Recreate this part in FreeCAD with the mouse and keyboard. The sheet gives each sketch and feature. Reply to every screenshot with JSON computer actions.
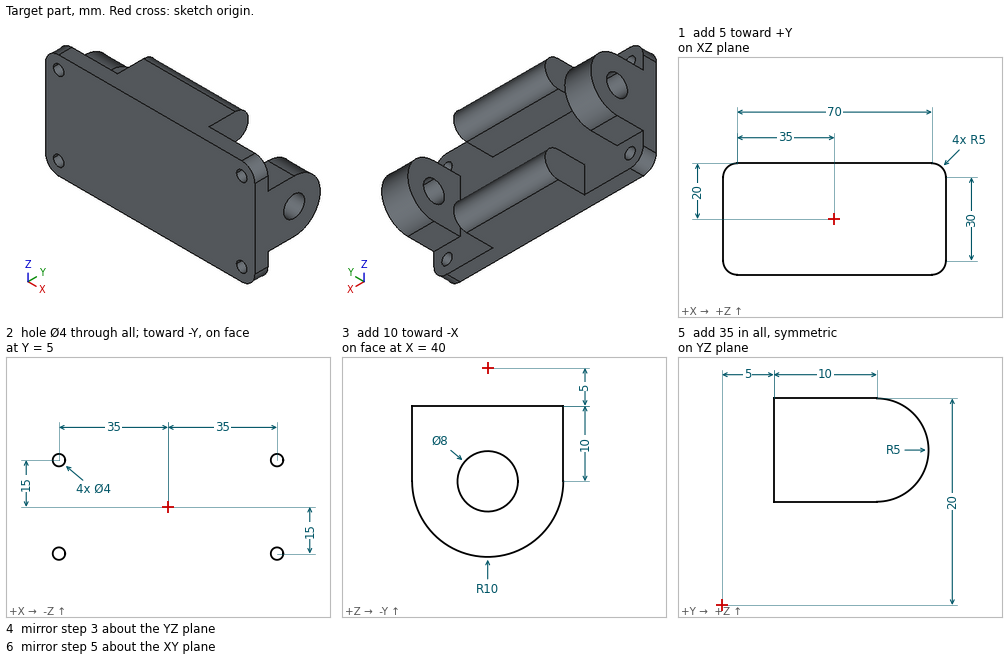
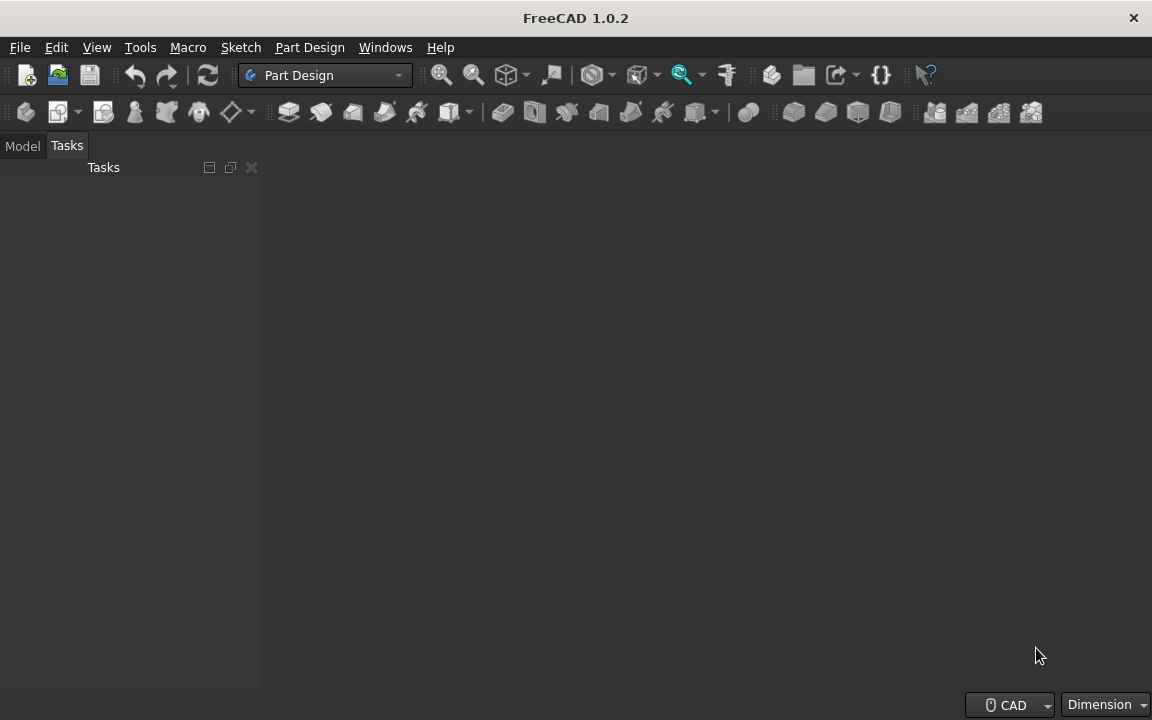
{"action": "left_click", "coordinate": [26, 76]}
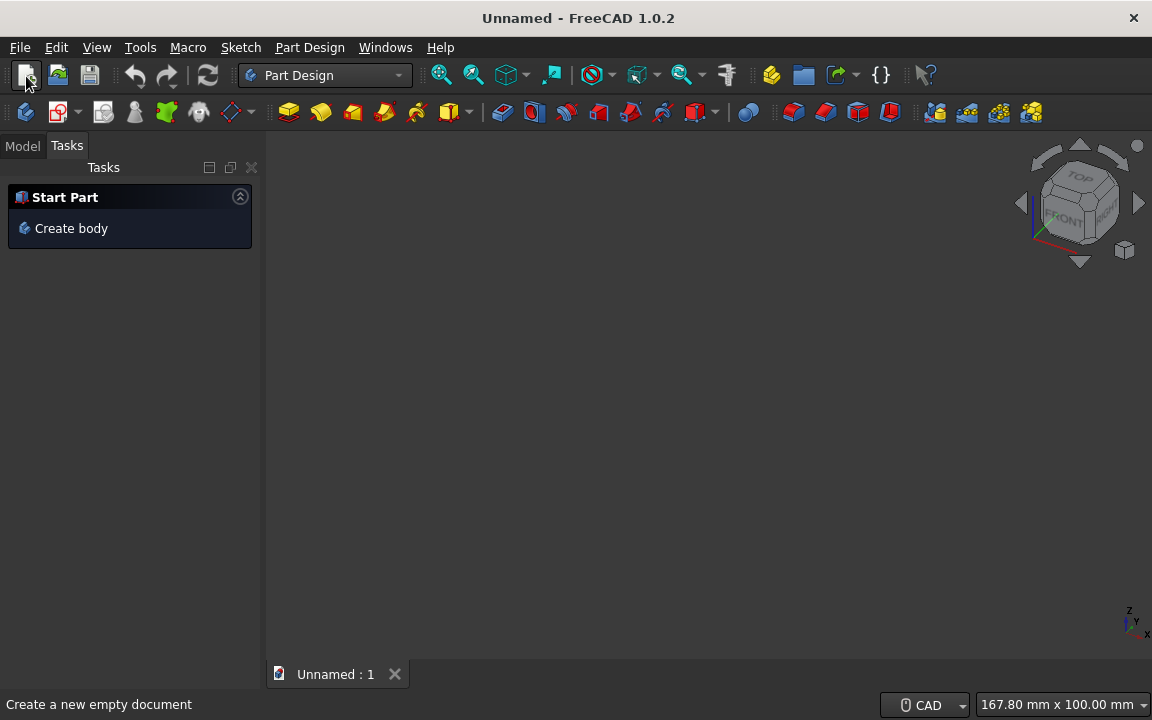
{"action": "left_click", "coordinate": [58, 112]}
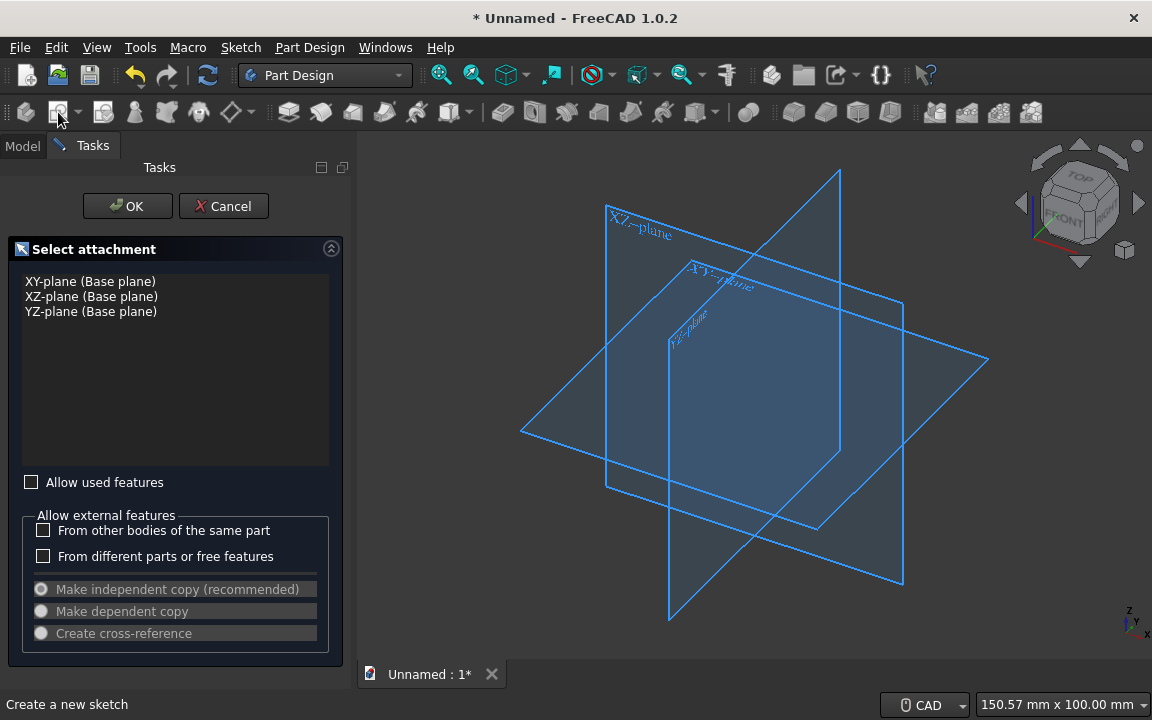
{"action": "left_click", "coordinate": [82, 296]}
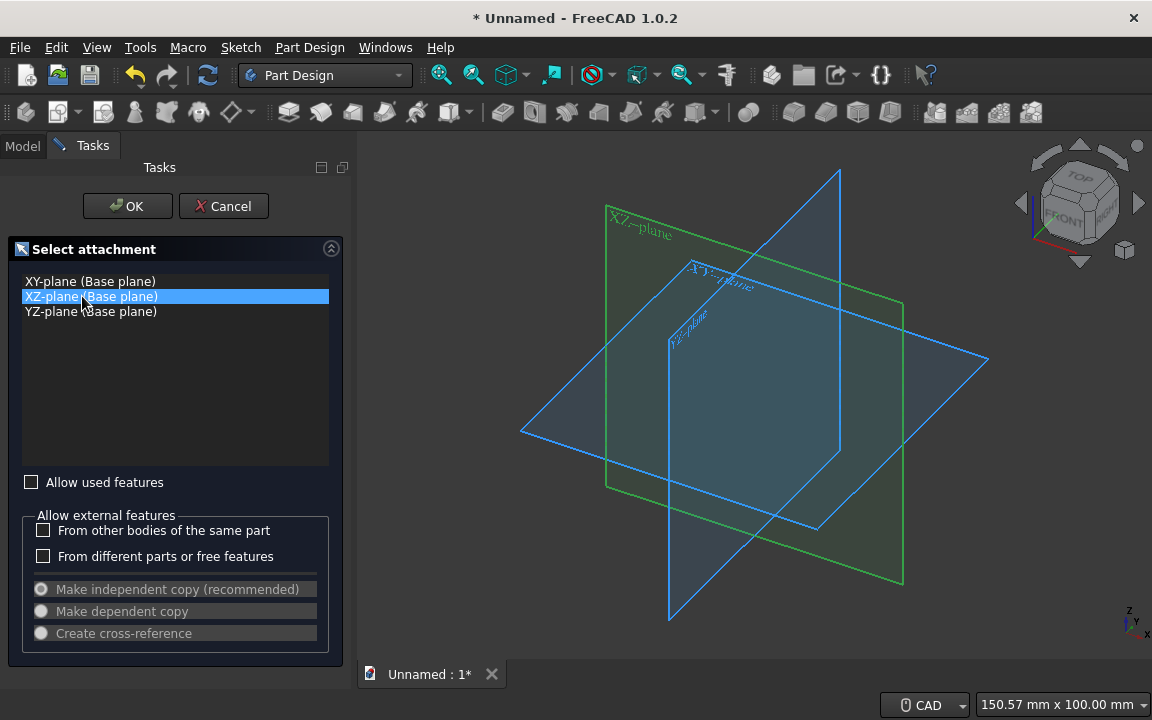
{"action": "left_click", "coordinate": [128, 206]}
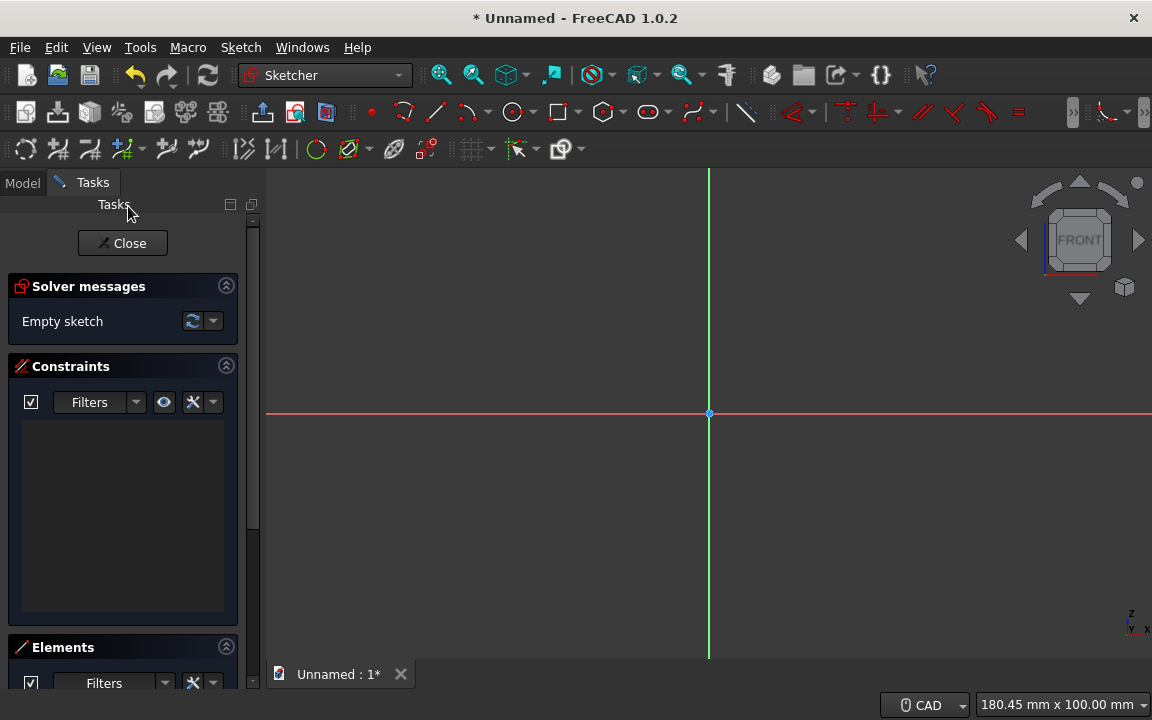
{"action": "left_click", "coordinate": [436, 112]}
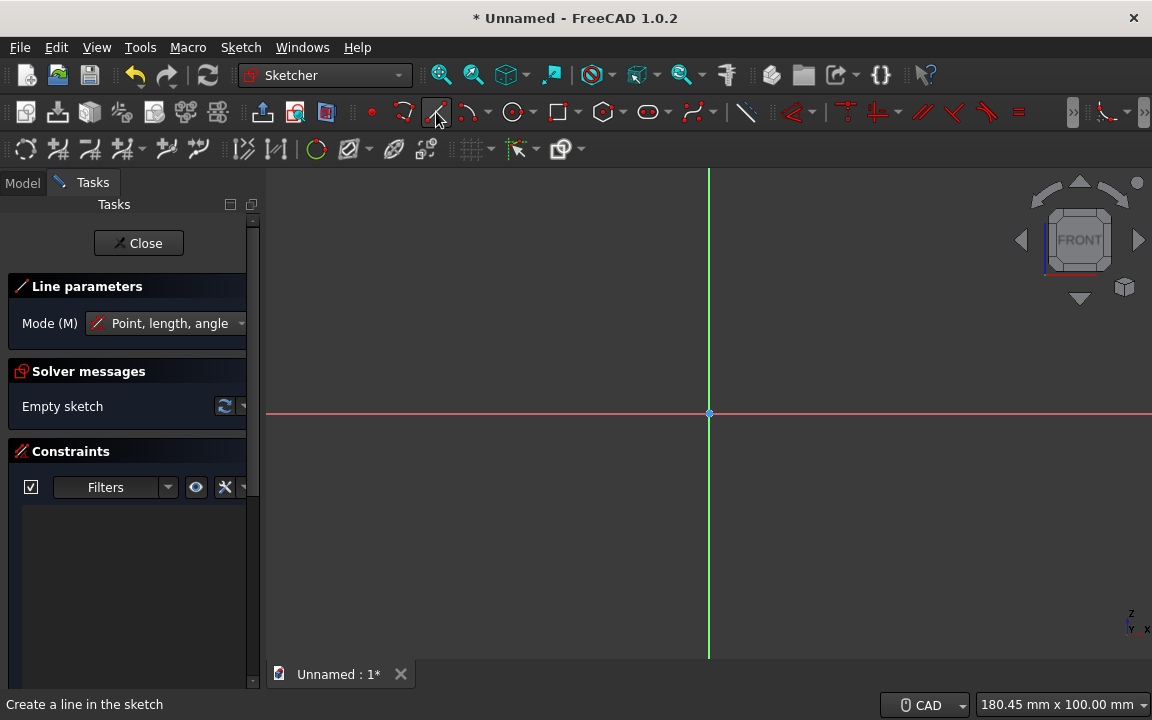
{"action": "left_click", "coordinate": [537, 315]}
{"action": "left_click", "coordinate": [881, 315]}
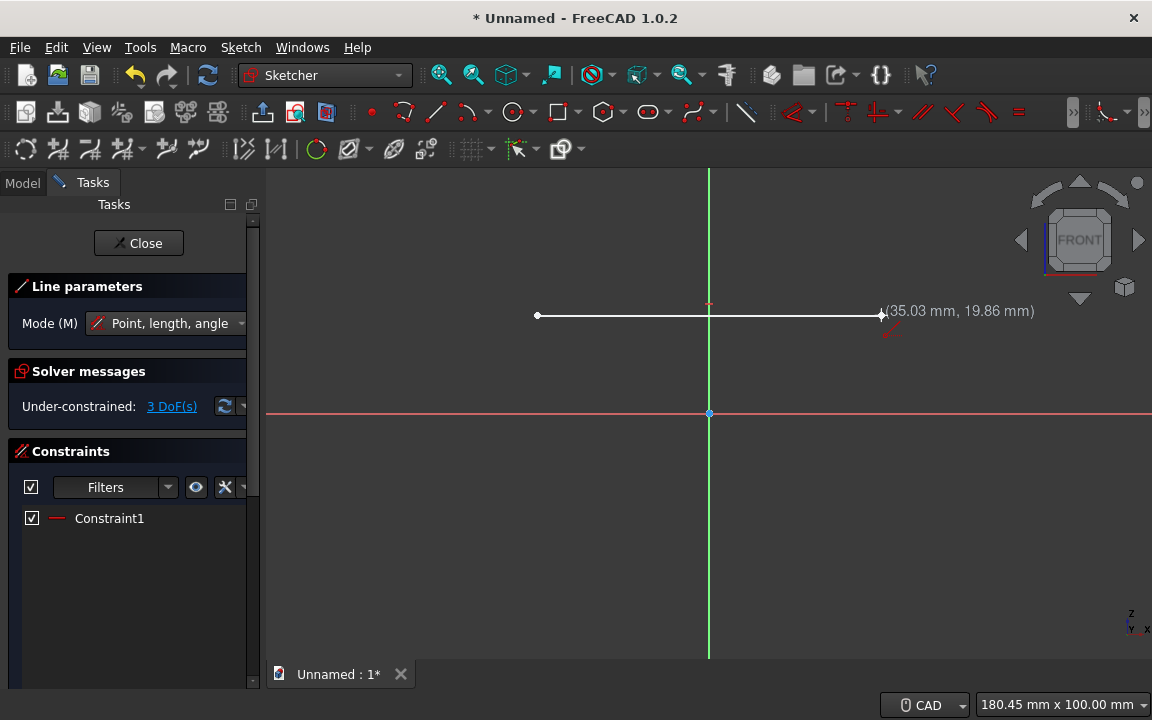
{"action": "left_click", "coordinate": [905, 340]}
{"action": "left_click", "coordinate": [905, 487]}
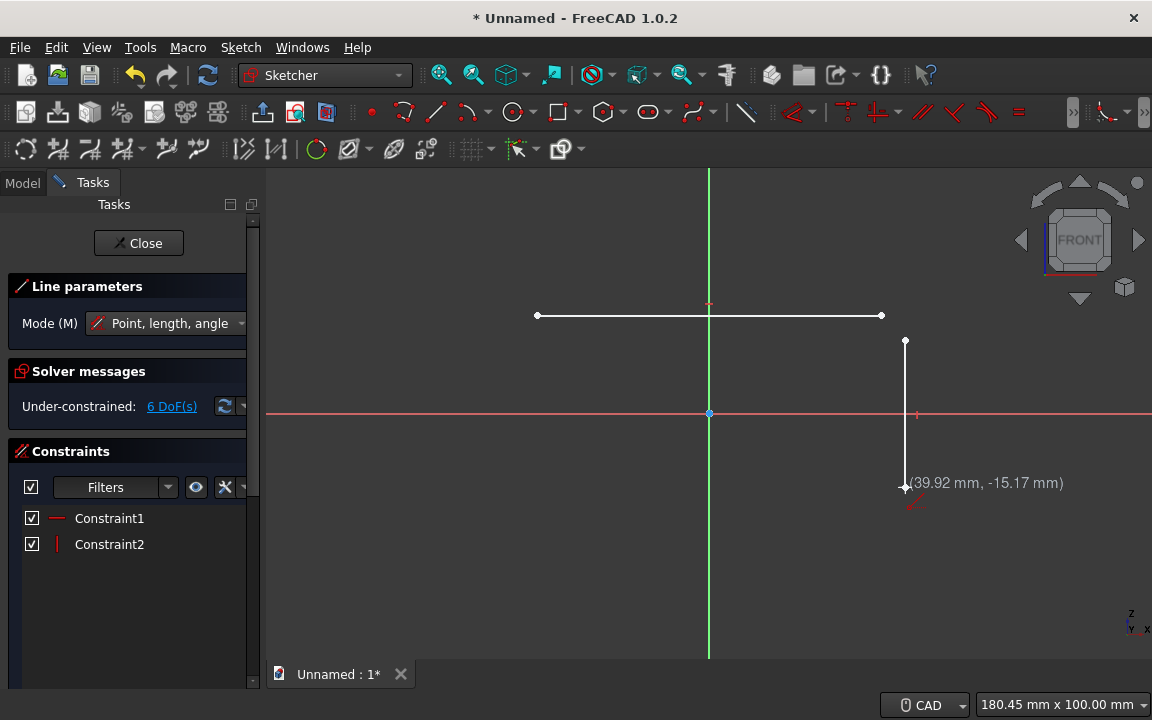
{"action": "left_click", "coordinate": [881, 512]}
{"action": "left_click", "coordinate": [537, 512]}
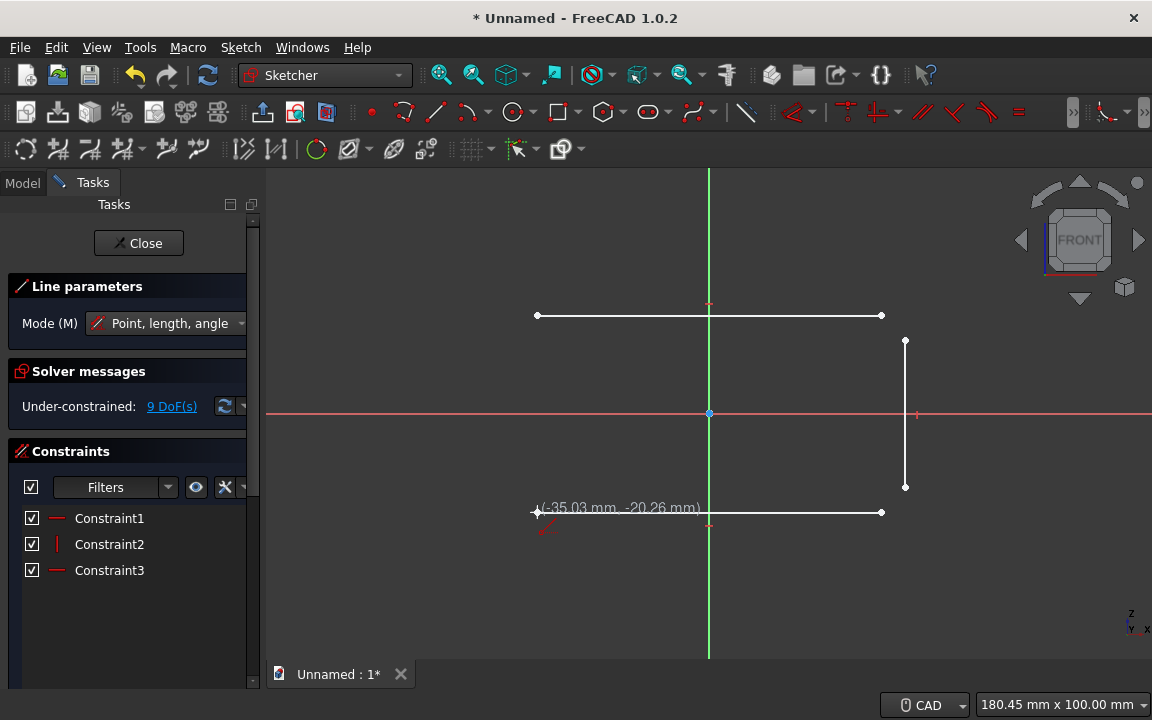
{"action": "left_click", "coordinate": [513, 487]}
{"action": "left_click", "coordinate": [513, 340]}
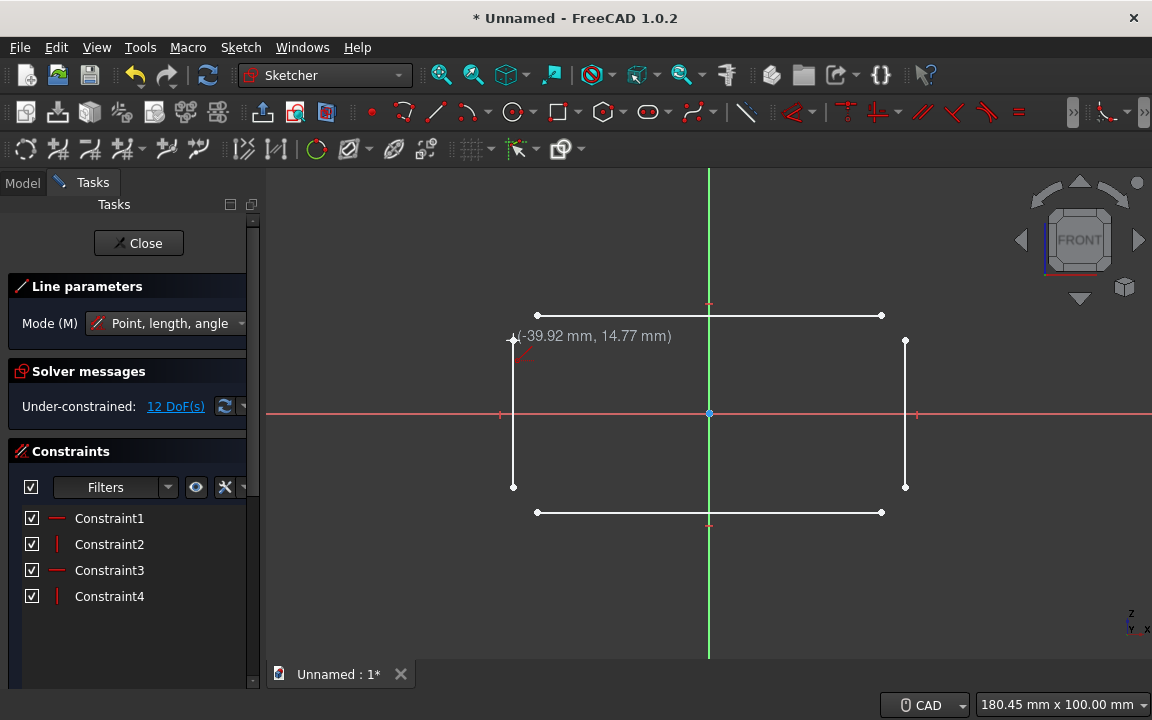
{"action": "key", "text": "g 3 a"}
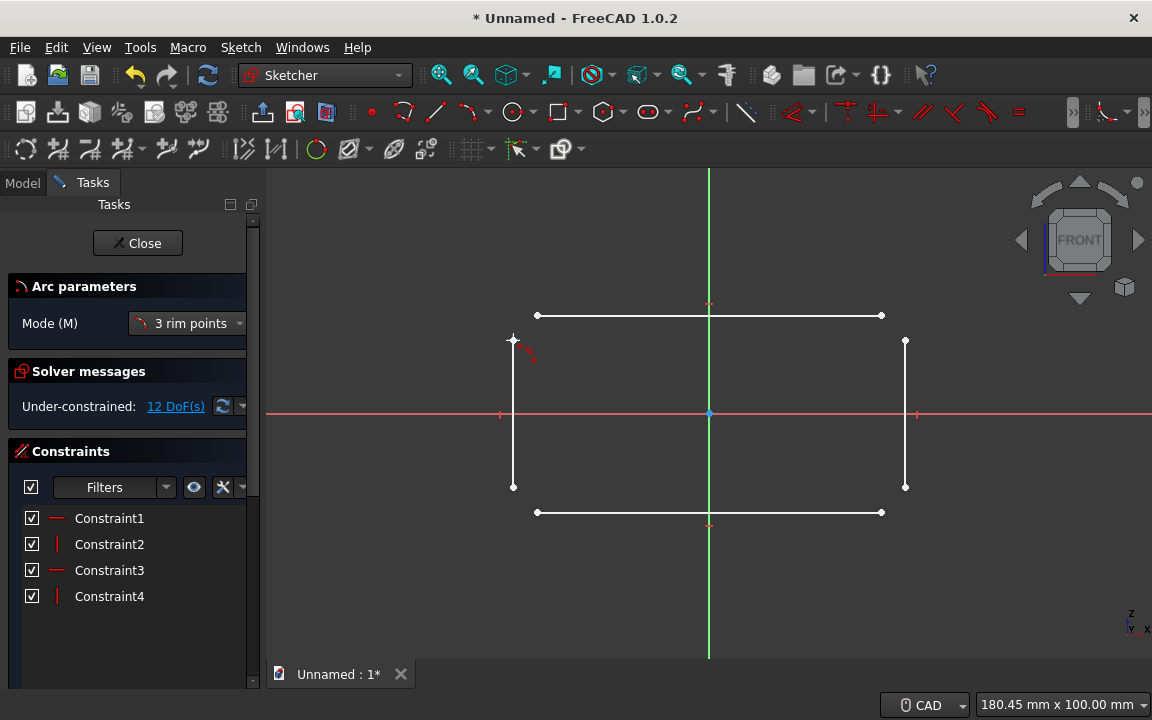
{"action": "left_click", "coordinate": [881, 316]}
{"action": "left_click", "coordinate": [905, 341]}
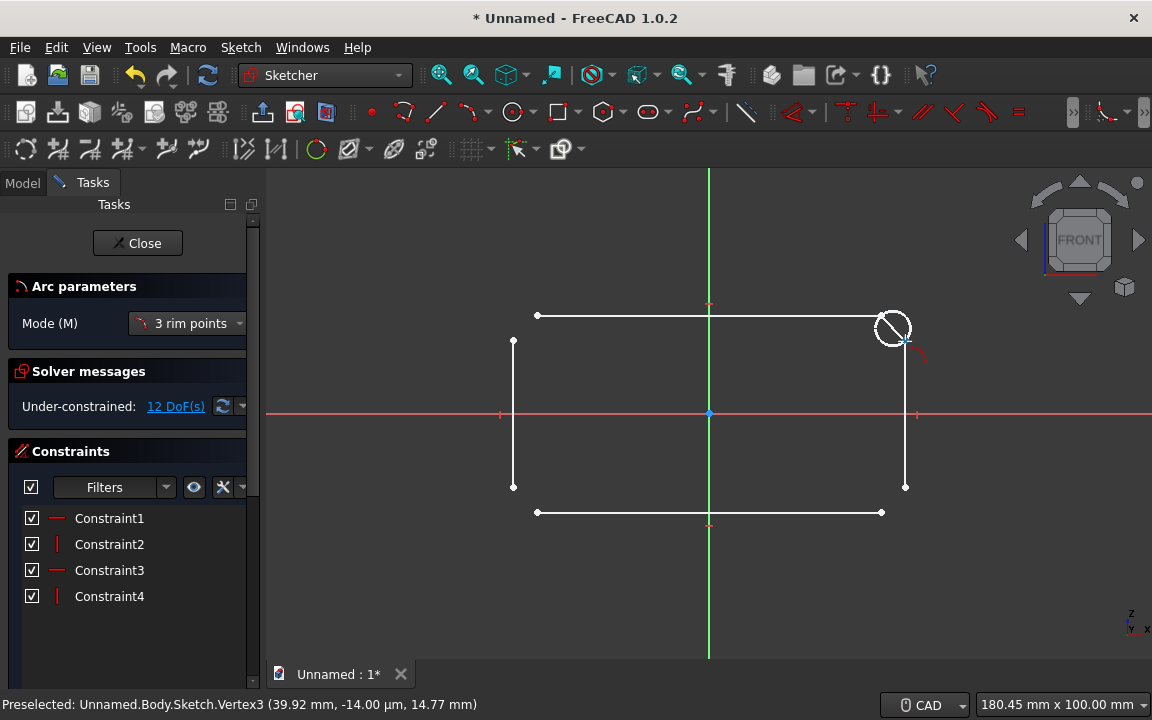
{"action": "scroll", "coordinate": [898, 322], "scroll_direction": "up", "scroll_amount": 4}